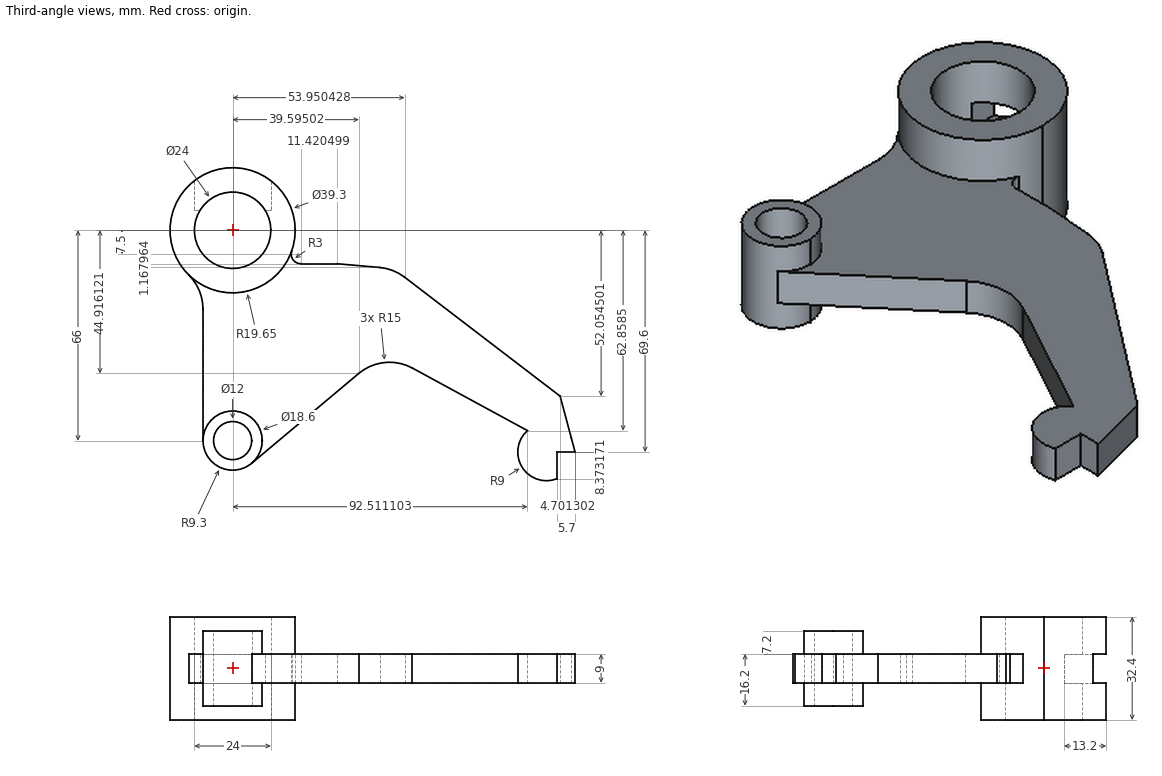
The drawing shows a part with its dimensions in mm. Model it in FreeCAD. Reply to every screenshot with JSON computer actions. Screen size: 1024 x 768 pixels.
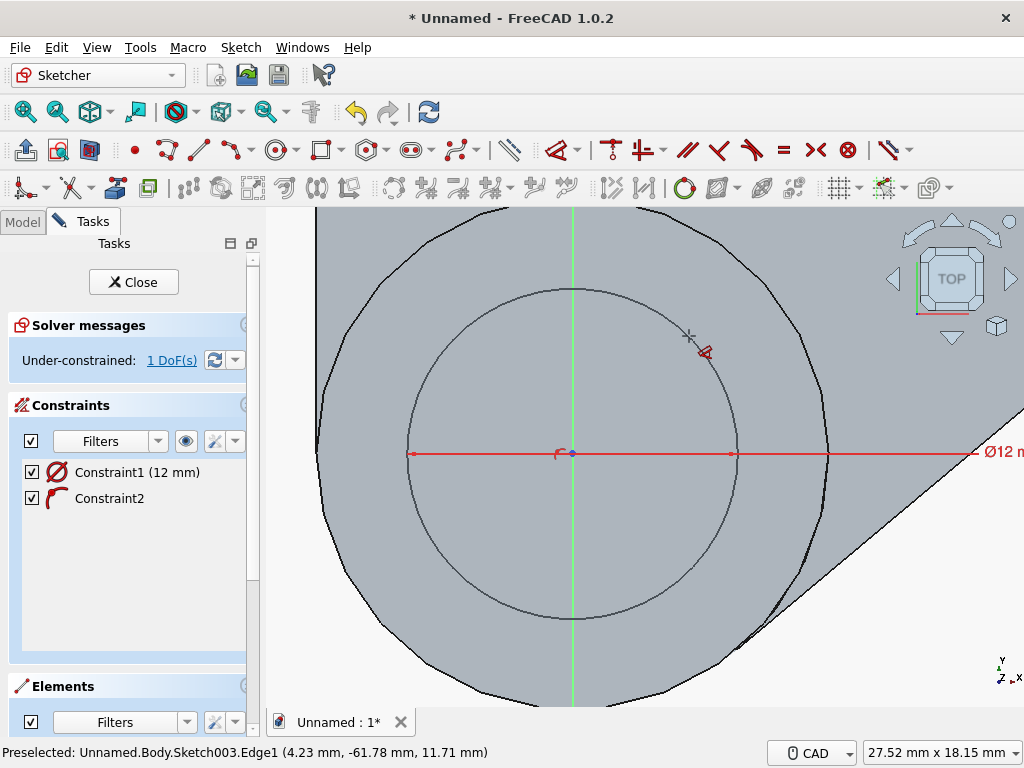
{"action": "left_click", "coordinate": [573, 454]}
{"action": "left_click", "coordinate": [607, 344]}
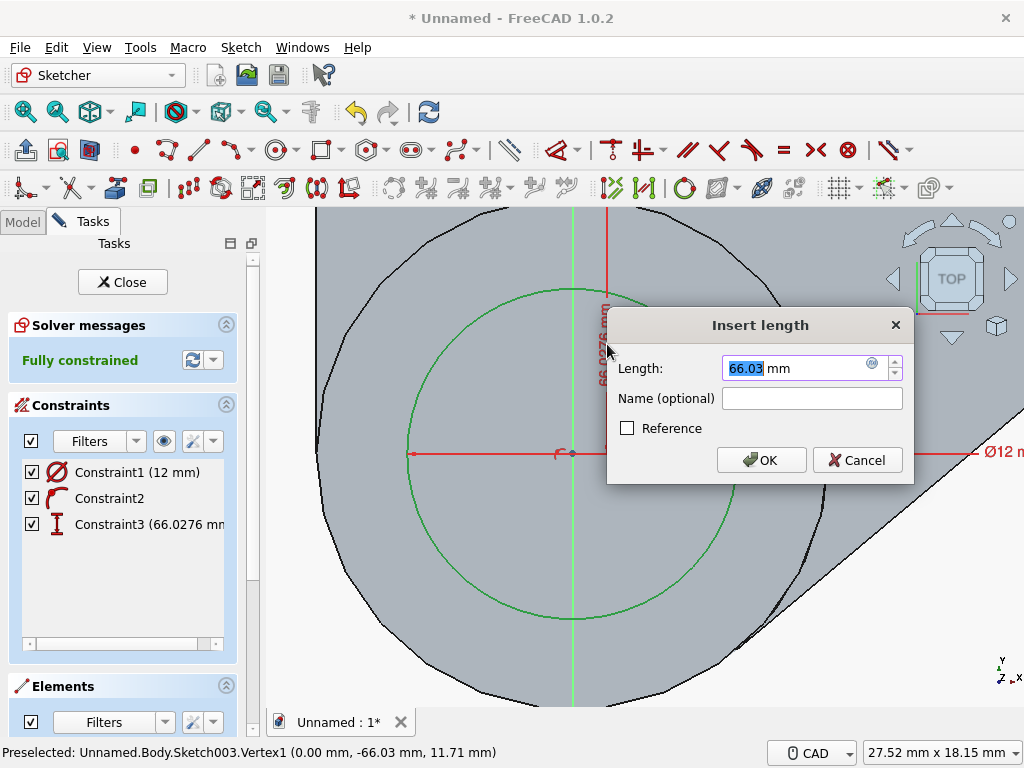
{"action": "type", "text": "66"}
{"action": "key", "text": "Return"}
{"action": "key", "text": "Escape"}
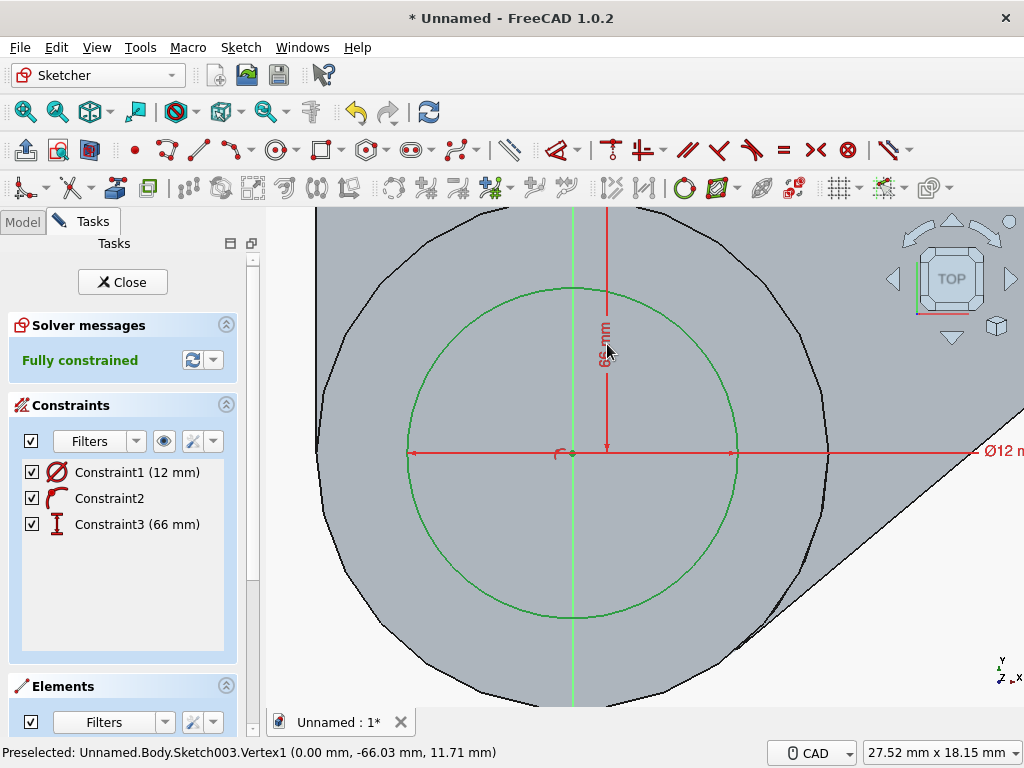
{"action": "left_click", "coordinate": [123, 282]}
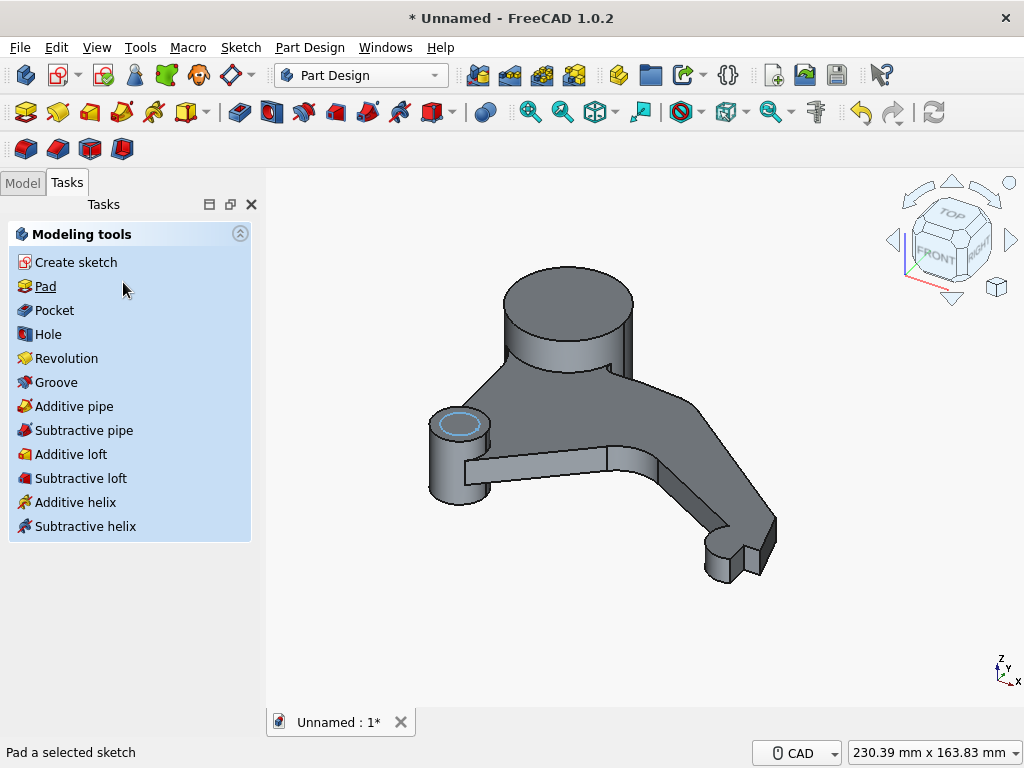
{"action": "left_click", "coordinate": [240, 112]}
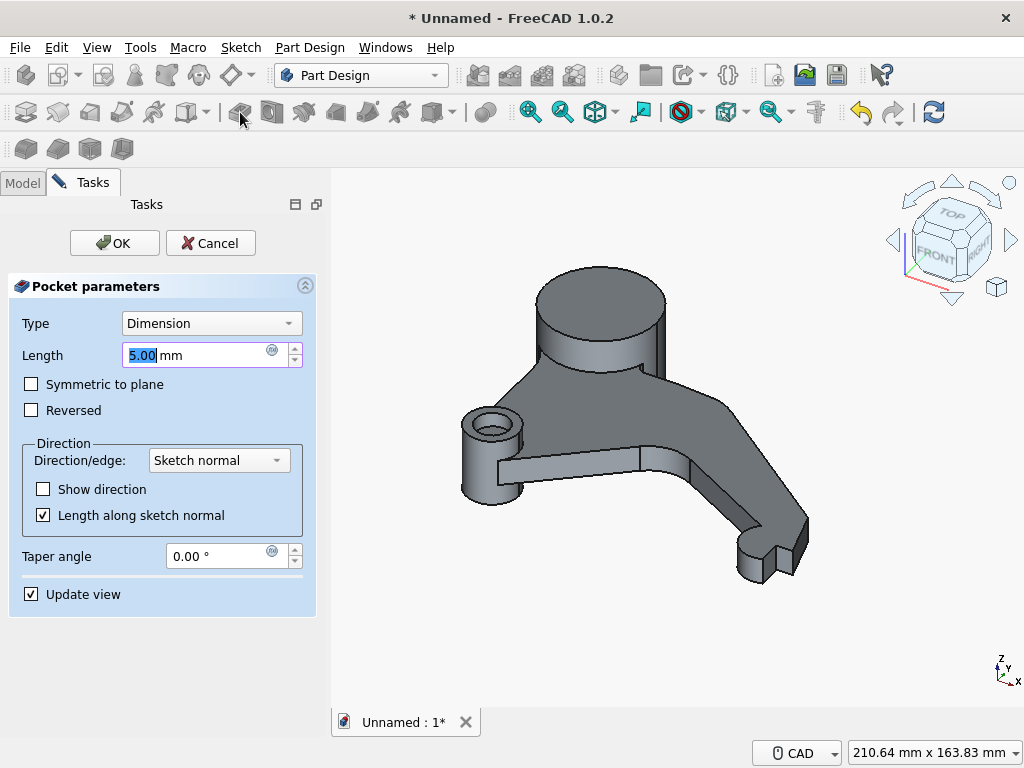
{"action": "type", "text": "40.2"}
{"action": "key", "text": "Tab"}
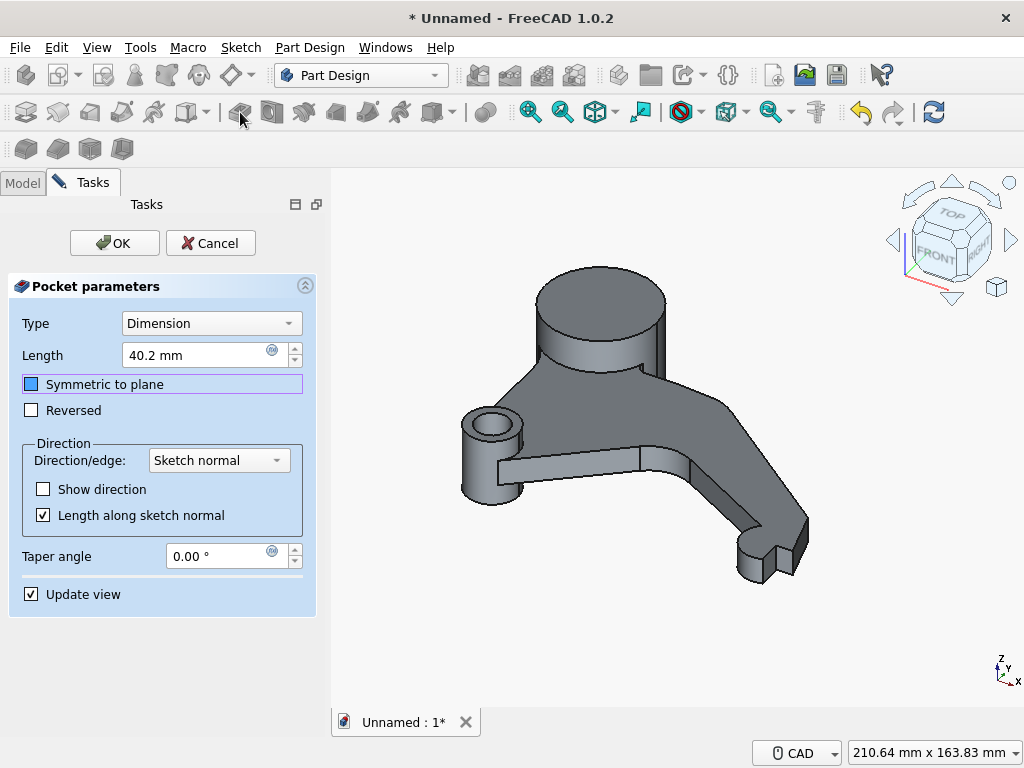
{"action": "left_click", "coordinate": [115, 243]}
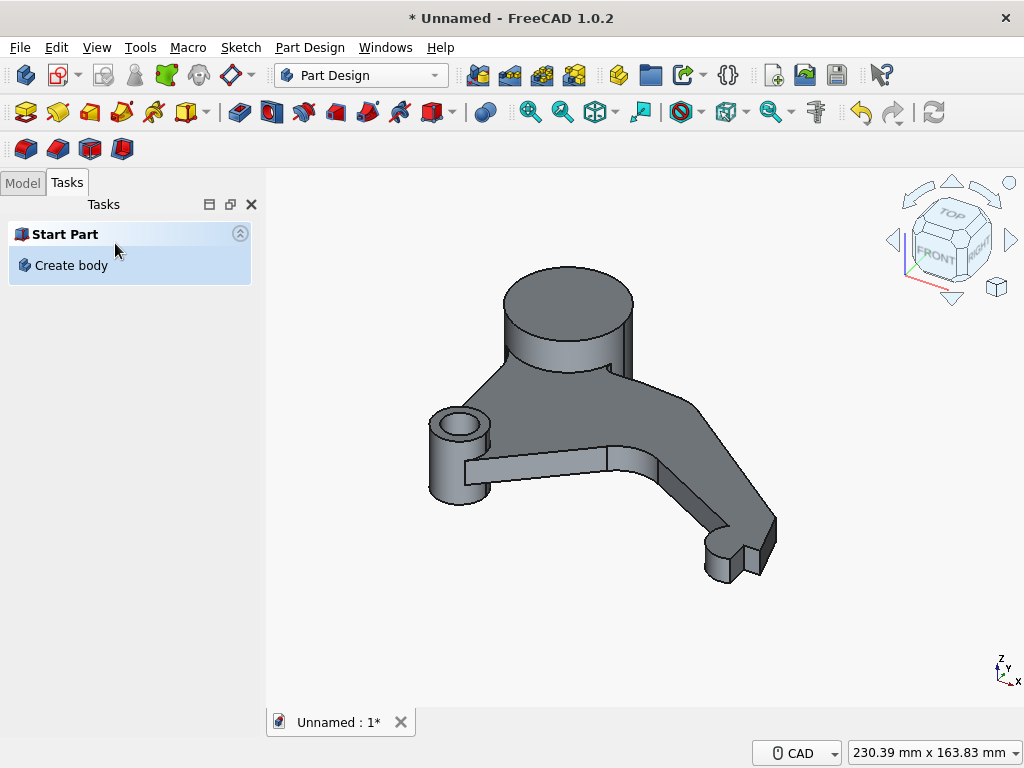
{"action": "left_click", "coordinate": [568, 303]}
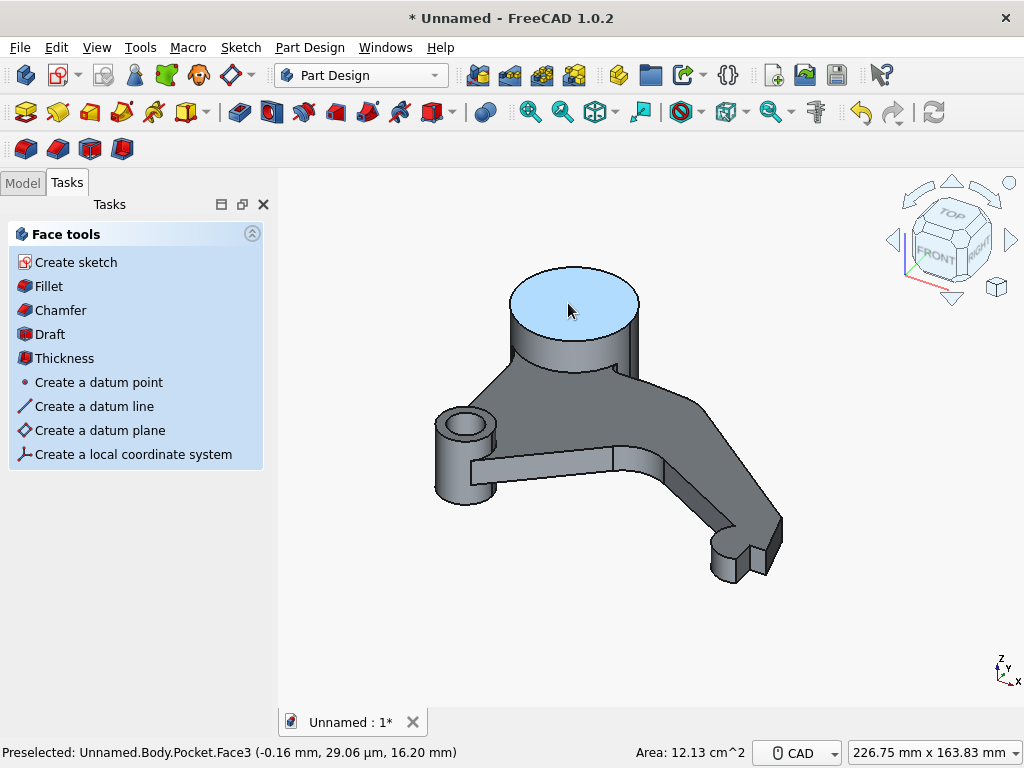
{"action": "left_click", "coordinate": [58, 76]}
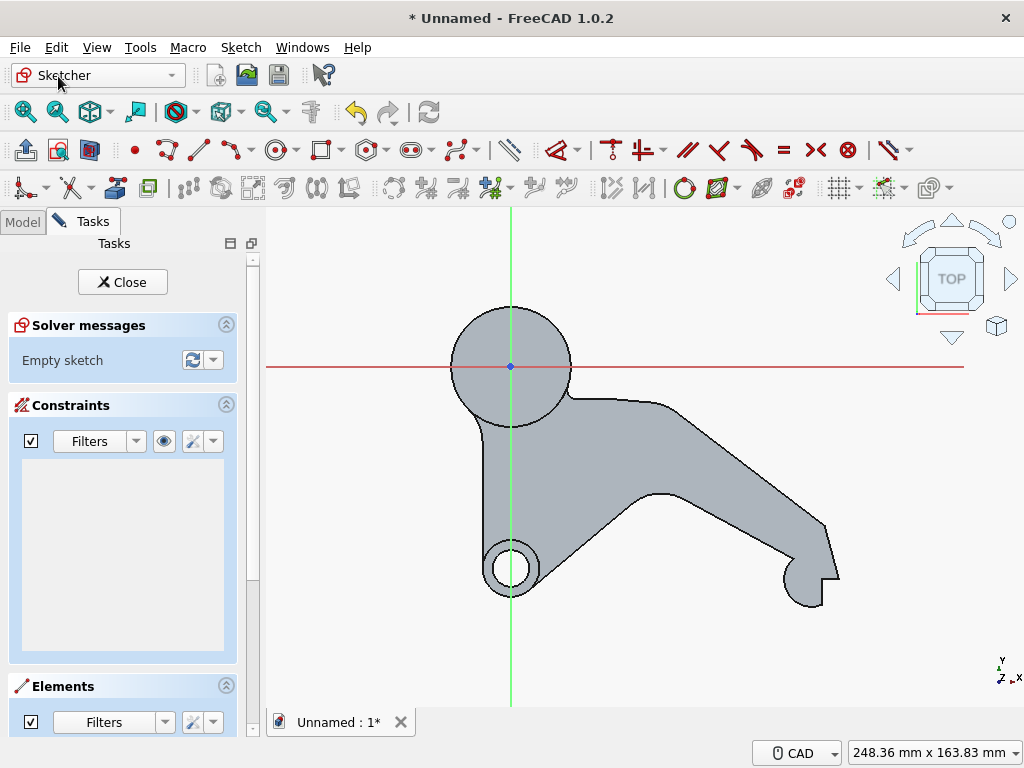
{"action": "scroll", "coordinate": [490, 338], "scroll_direction": "up", "scroll_amount": 7}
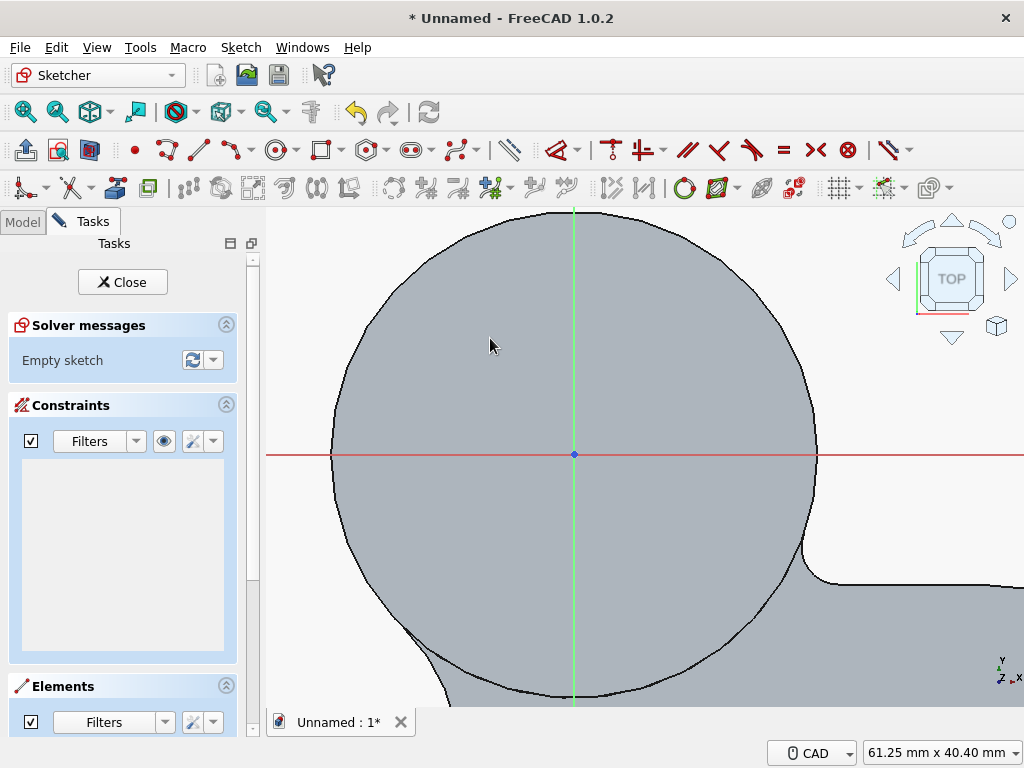
{"action": "left_click", "coordinate": [276, 150]}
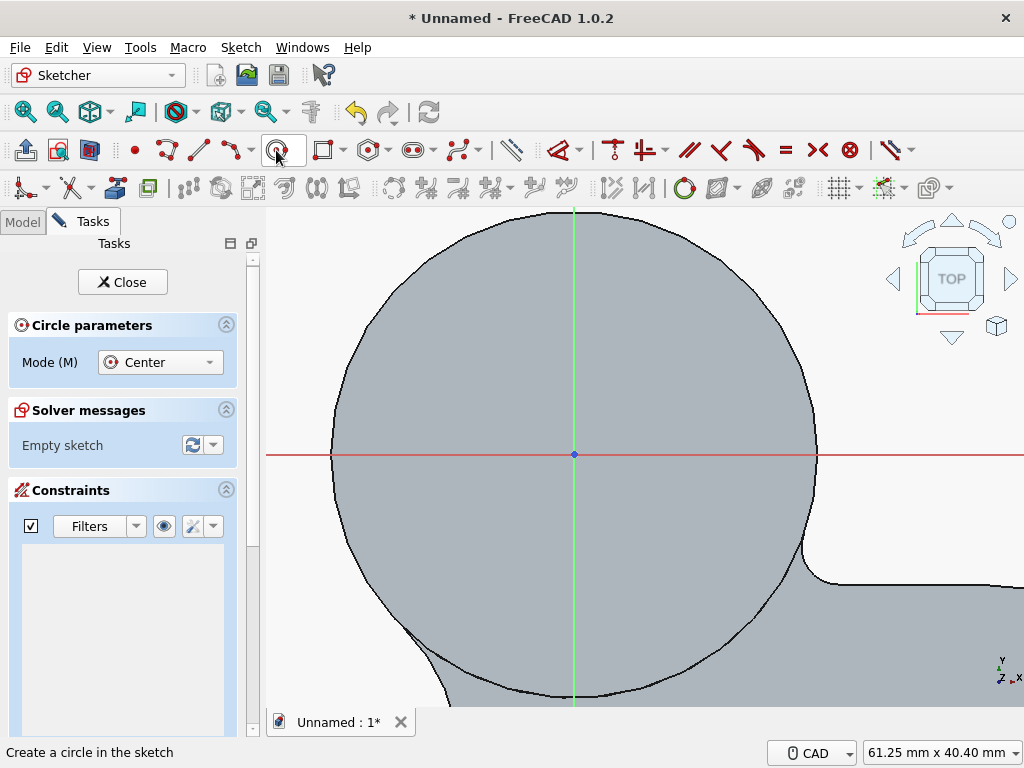
{"action": "left_click", "coordinate": [574, 455]}
{"action": "mouse_move", "coordinate": [679, 350]}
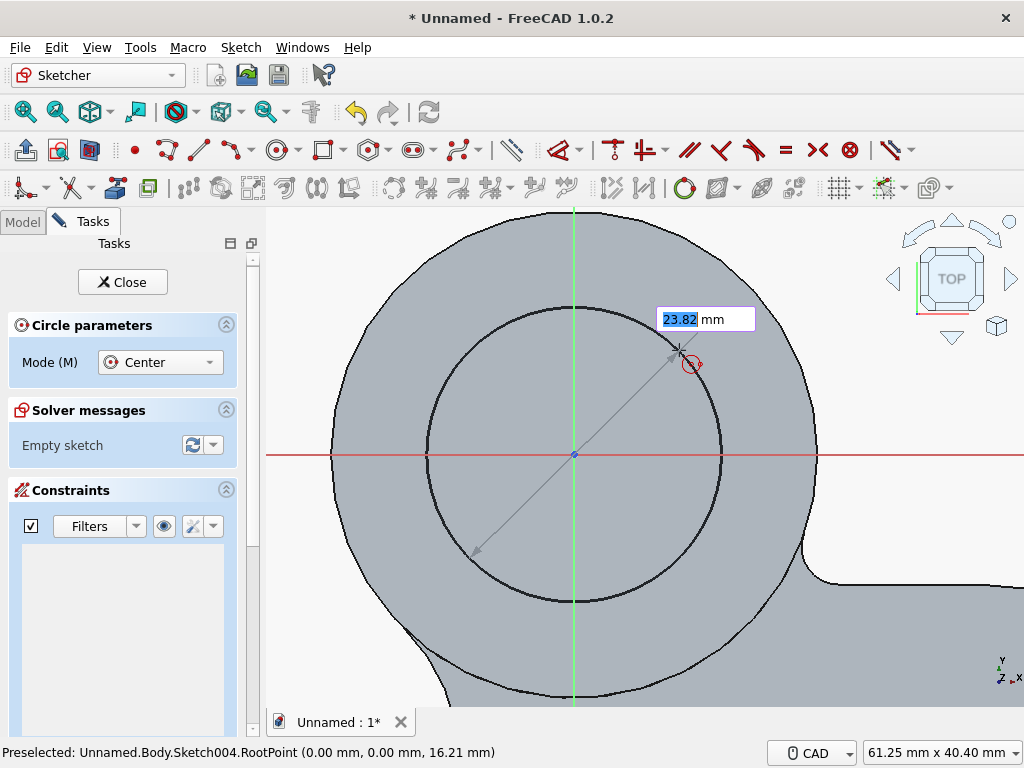
{"action": "type", "text": "24"}
{"action": "key", "text": "Return"}
{"action": "key", "text": "Escape"}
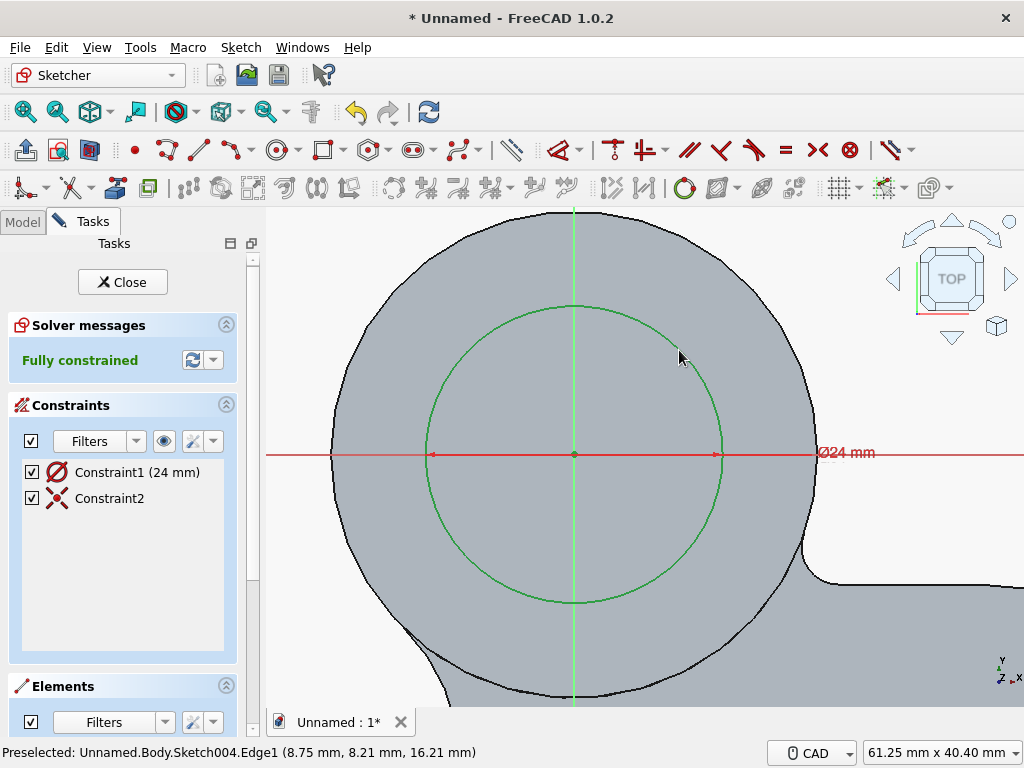
{"action": "left_click", "coordinate": [123, 282]}